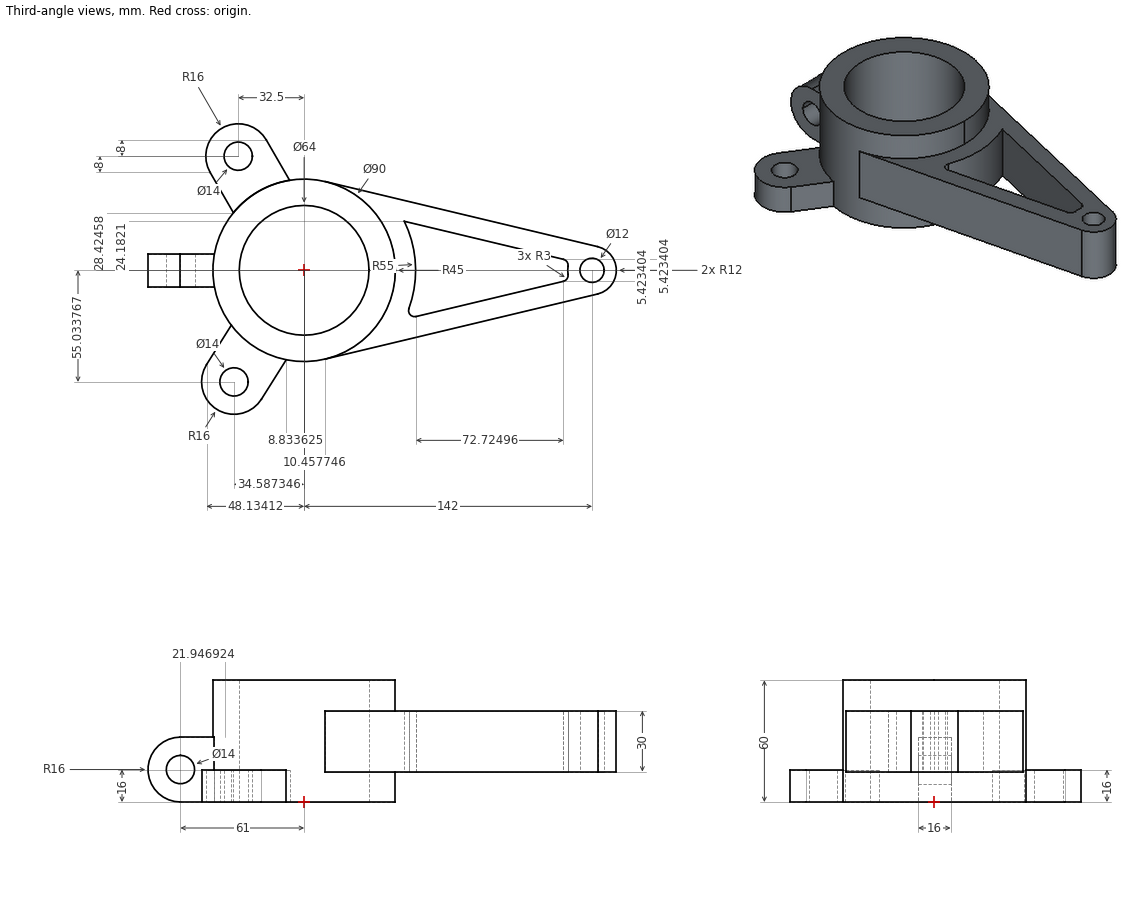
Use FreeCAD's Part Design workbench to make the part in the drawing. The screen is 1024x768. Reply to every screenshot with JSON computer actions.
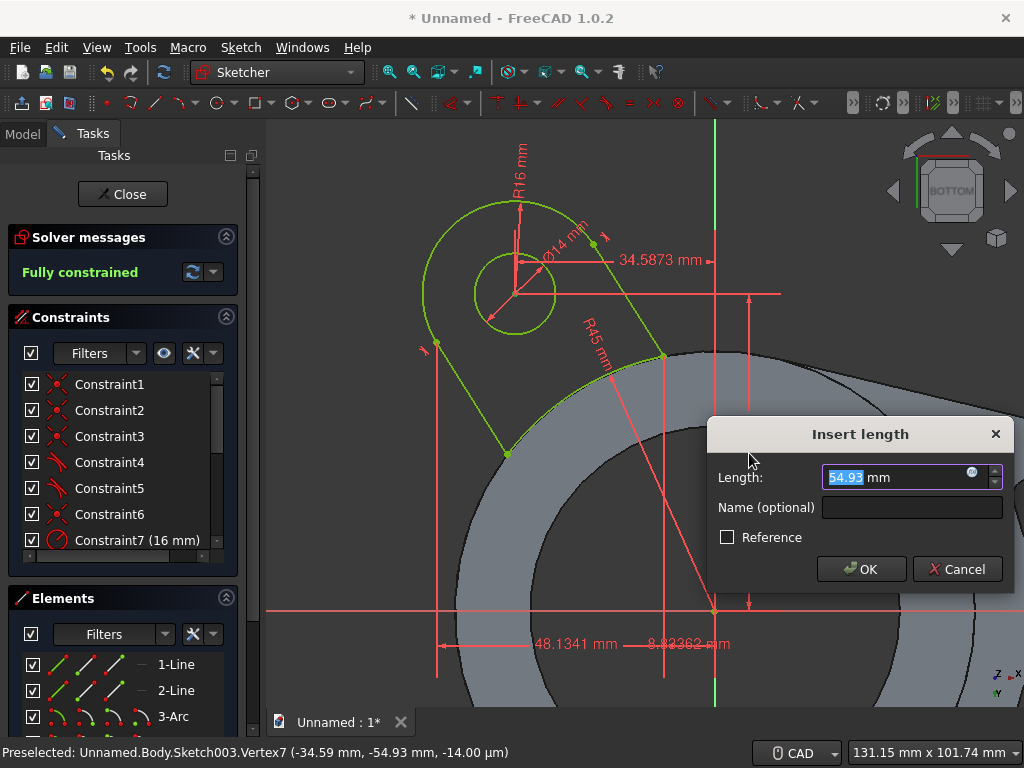
{"action": "type", "text": "55.033767"}
{"action": "key", "text": "Return"}
{"action": "key", "text": "Escape"}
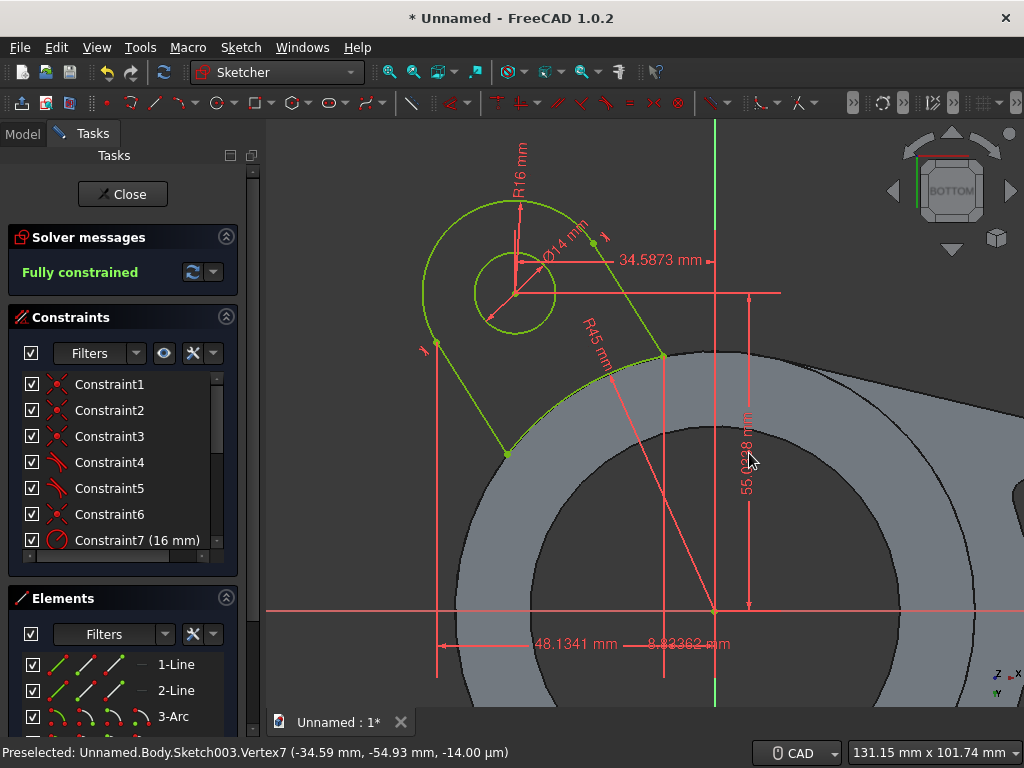
{"action": "left_click", "coordinate": [123, 194]}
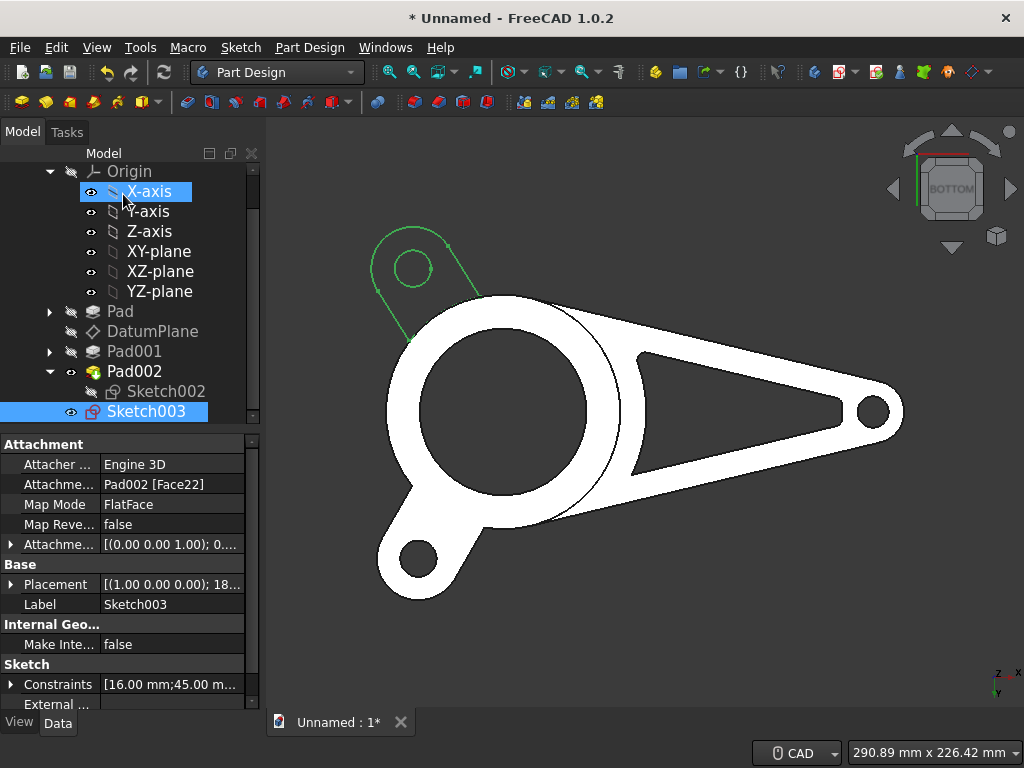
{"action": "left_click", "coordinate": [22, 102]}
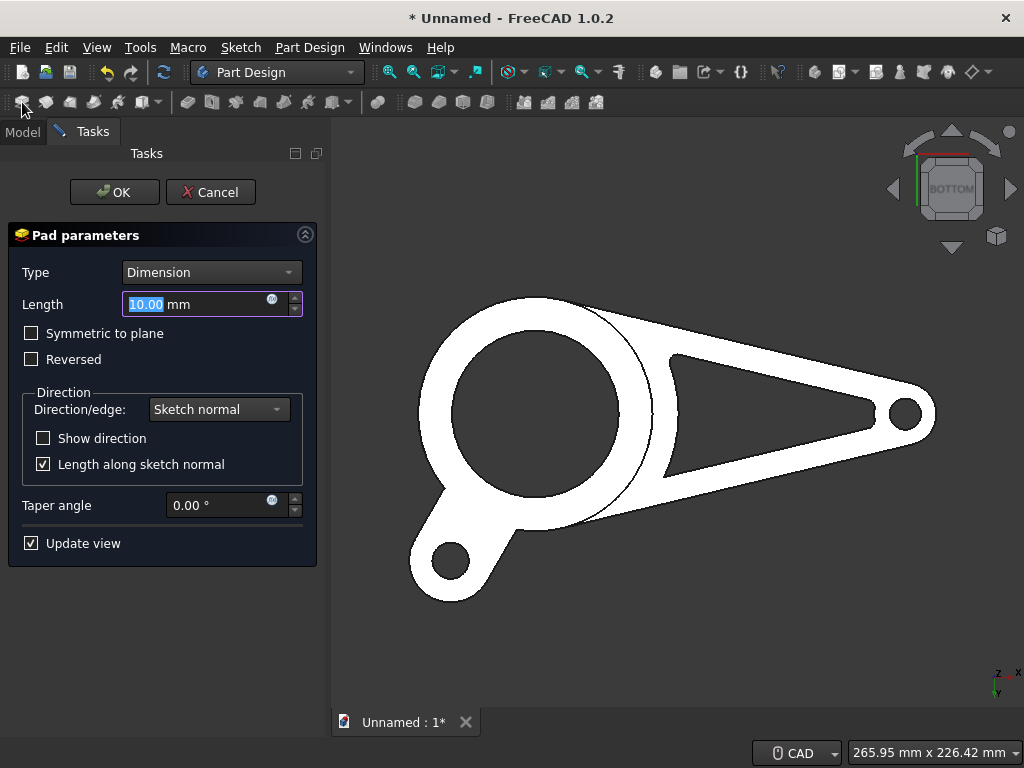
{"action": "type", "text": "16"}
{"action": "key", "text": "Tab"}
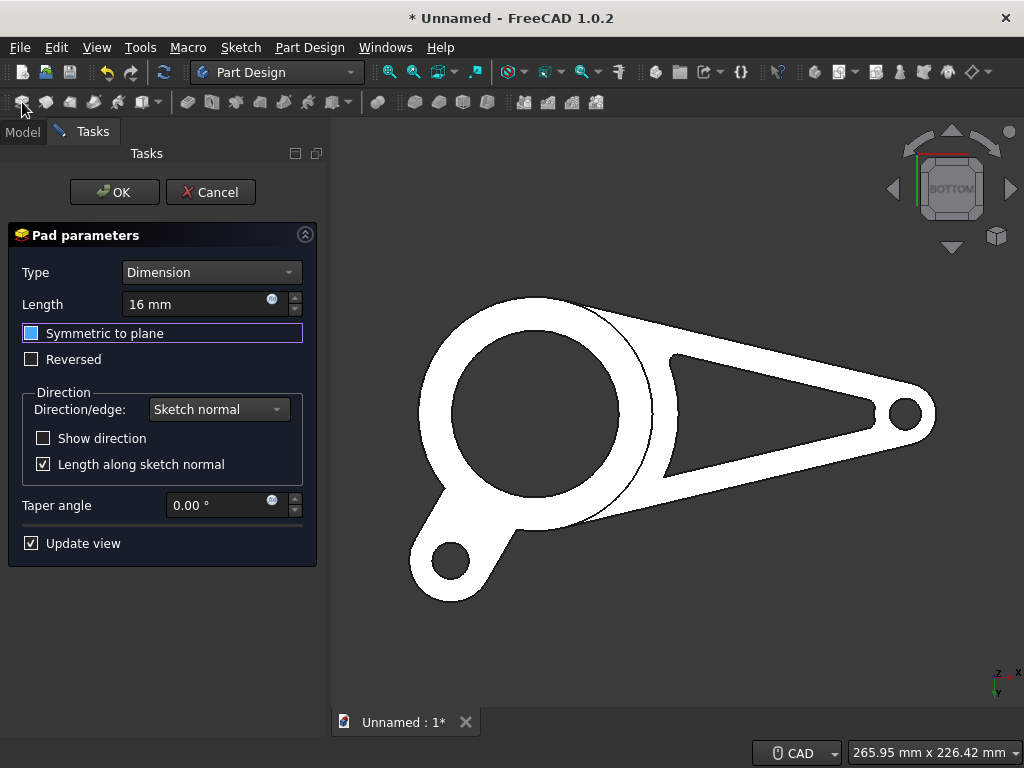
{"action": "left_click", "coordinate": [30, 359]}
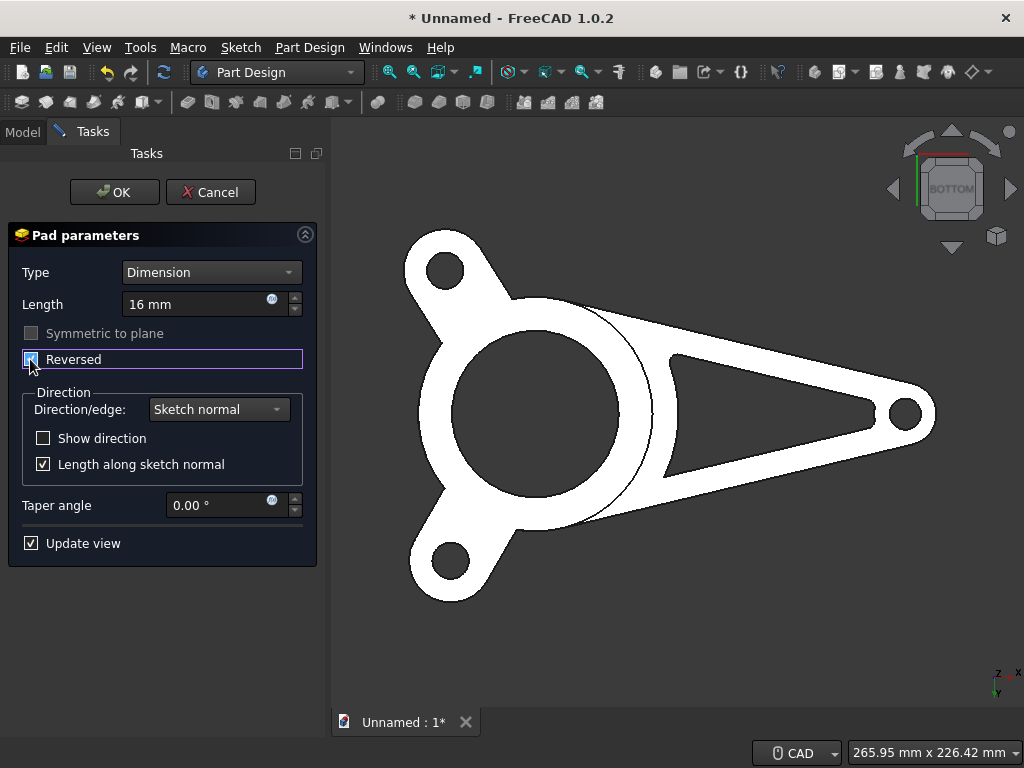
{"action": "left_click", "coordinate": [115, 192]}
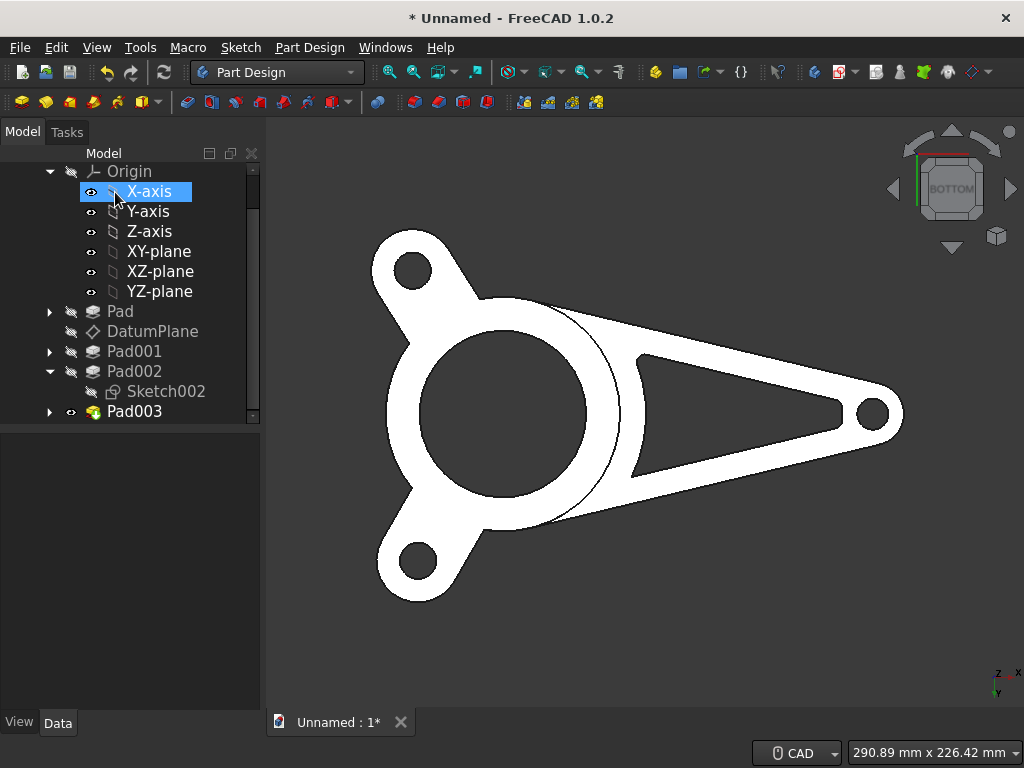
{"action": "left_click", "coordinate": [840, 72]}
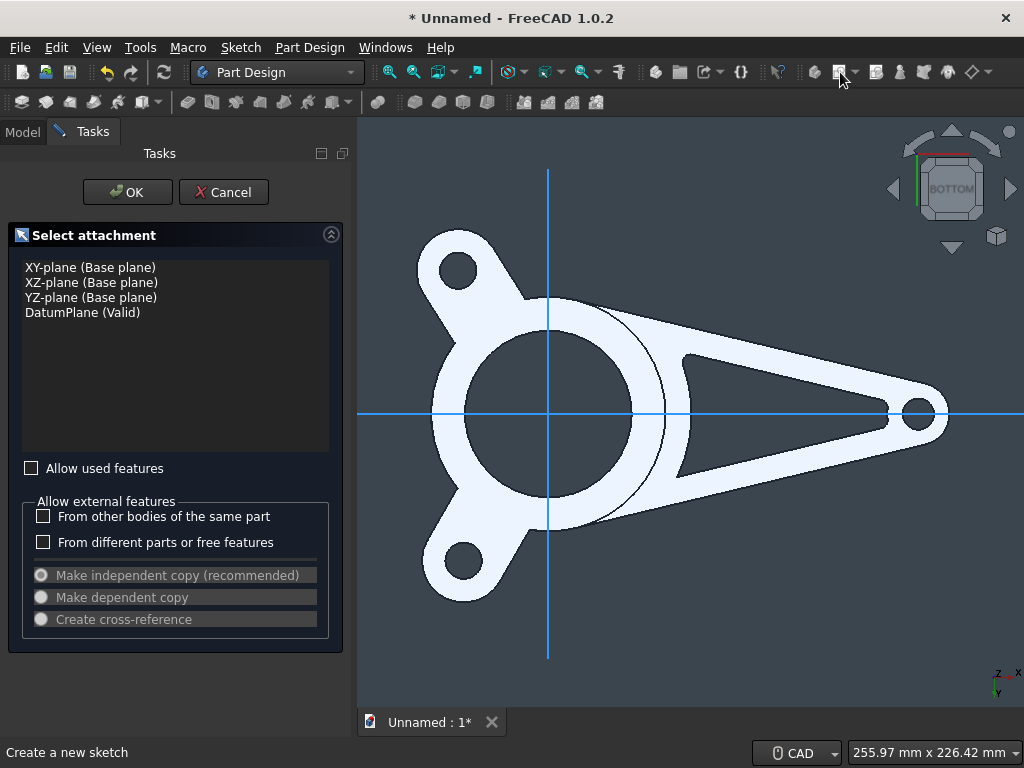
{"action": "left_click", "coordinate": [82, 282]}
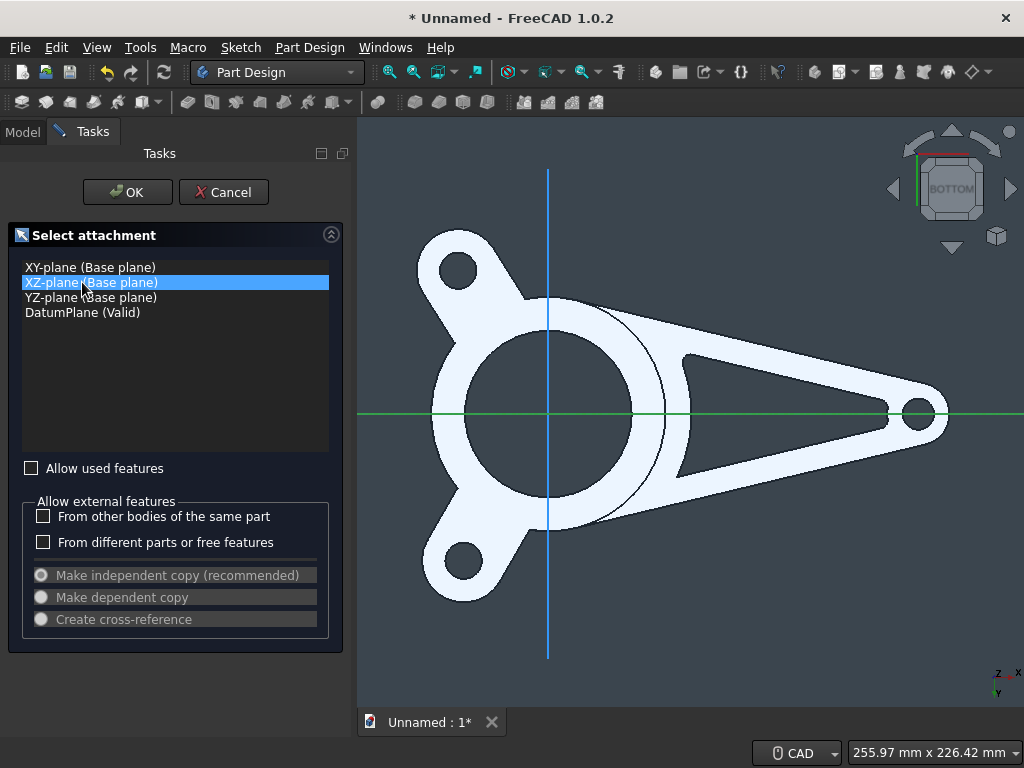
{"action": "left_click", "coordinate": [128, 192]}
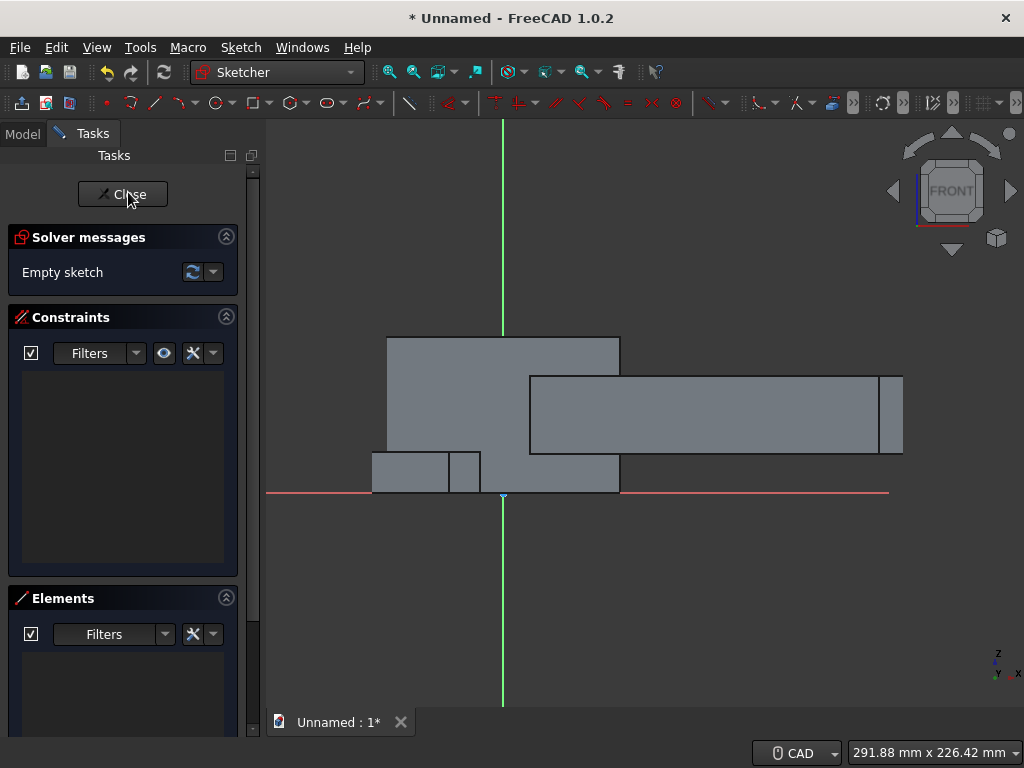
{"action": "left_click", "coordinate": [70, 104]}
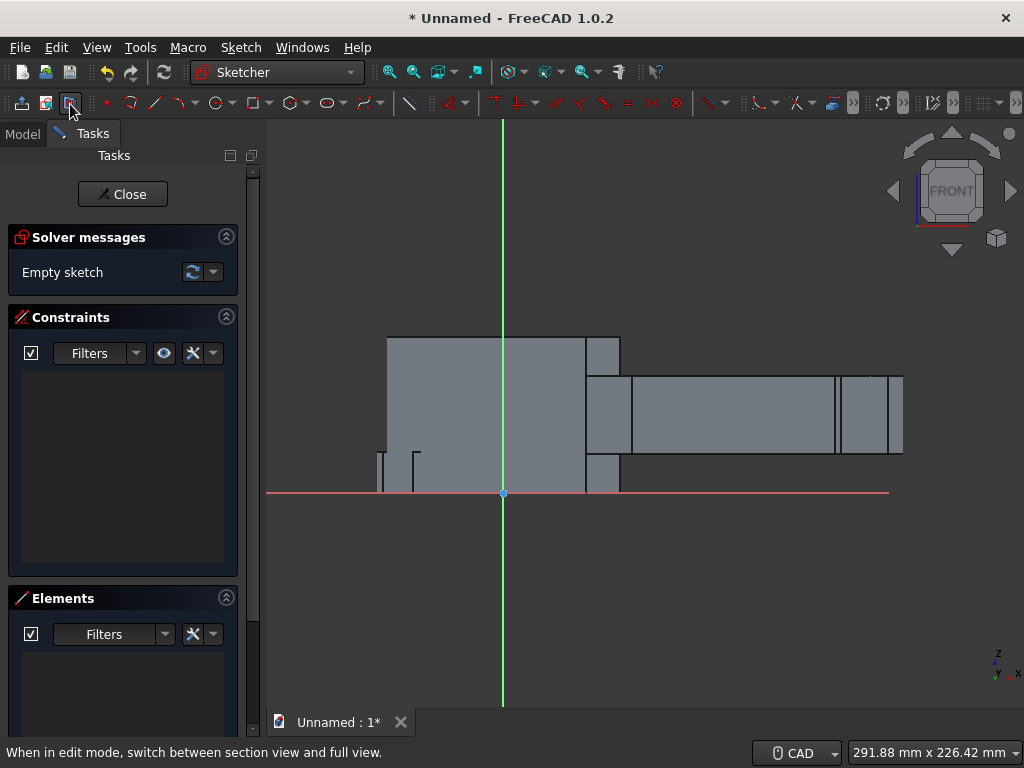
{"action": "scroll", "coordinate": [576, 413], "scroll_direction": "down", "scroll_amount": 5}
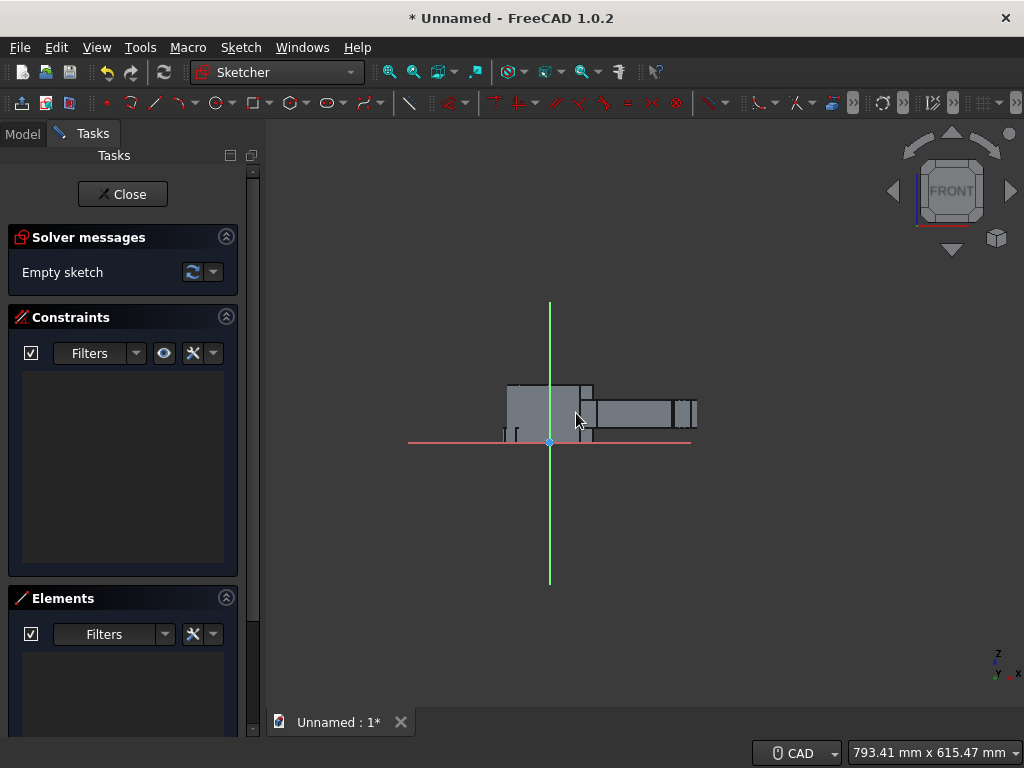
{"action": "scroll", "coordinate": [497, 431], "scroll_direction": "up", "scroll_amount": 8}